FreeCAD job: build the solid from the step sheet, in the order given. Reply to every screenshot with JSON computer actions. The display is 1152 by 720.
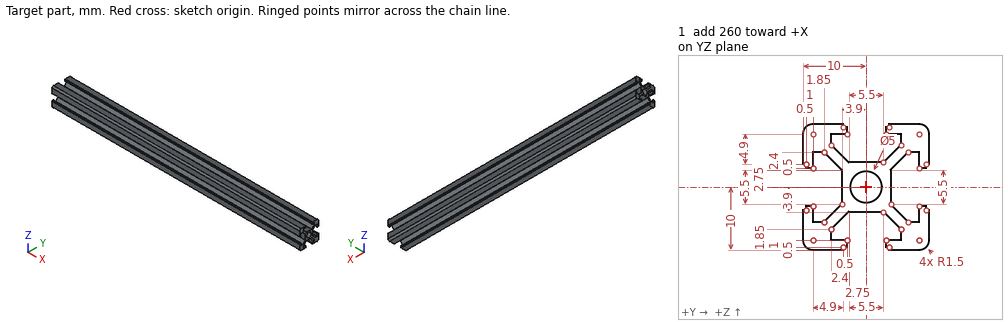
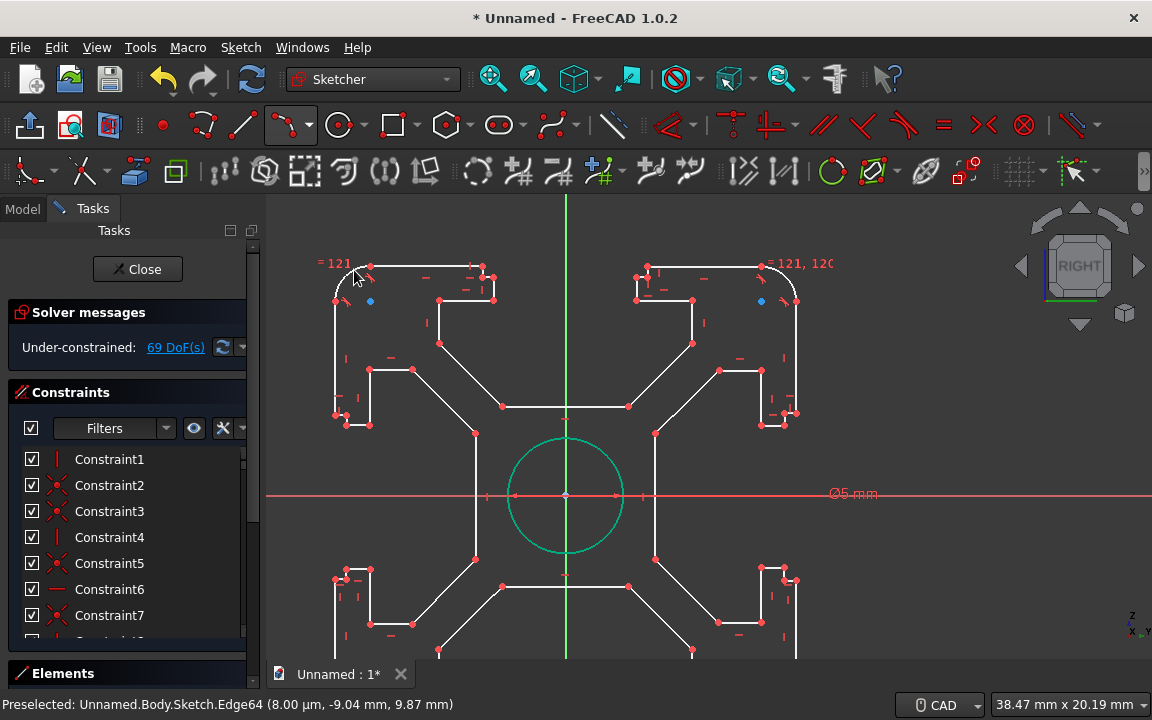
{"action": "scroll", "coordinate": [793, 286], "scroll_direction": "down", "scroll_amount": 2}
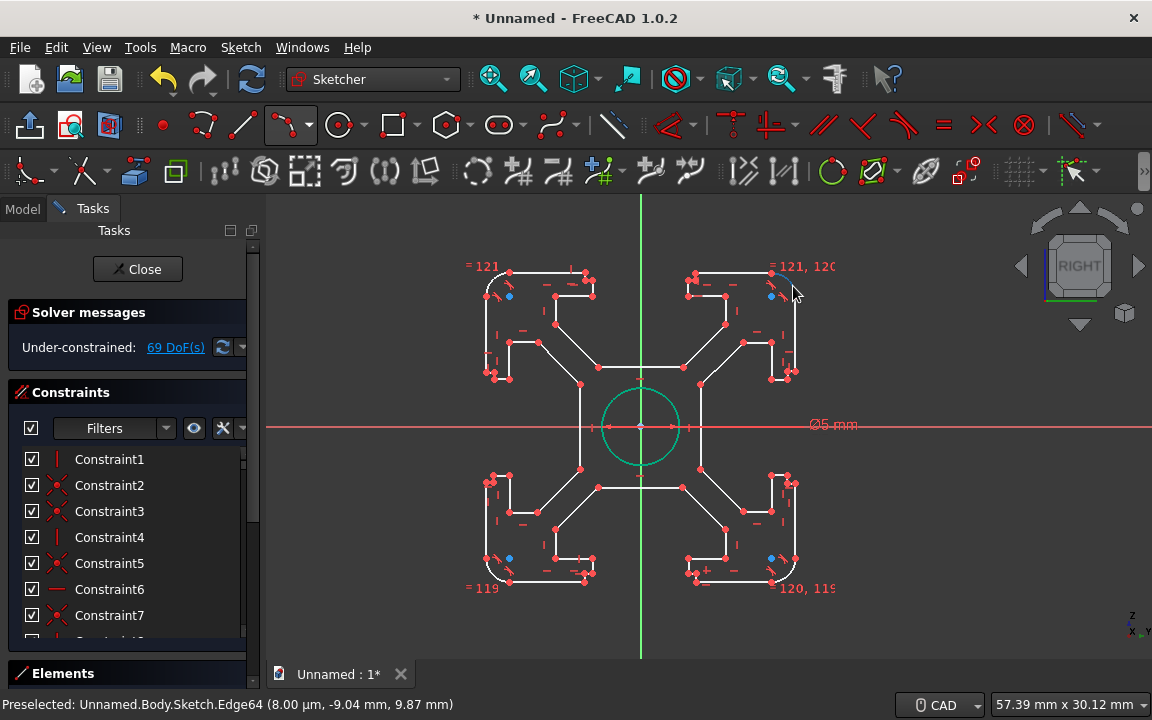
{"action": "left_click", "coordinate": [510, 559]}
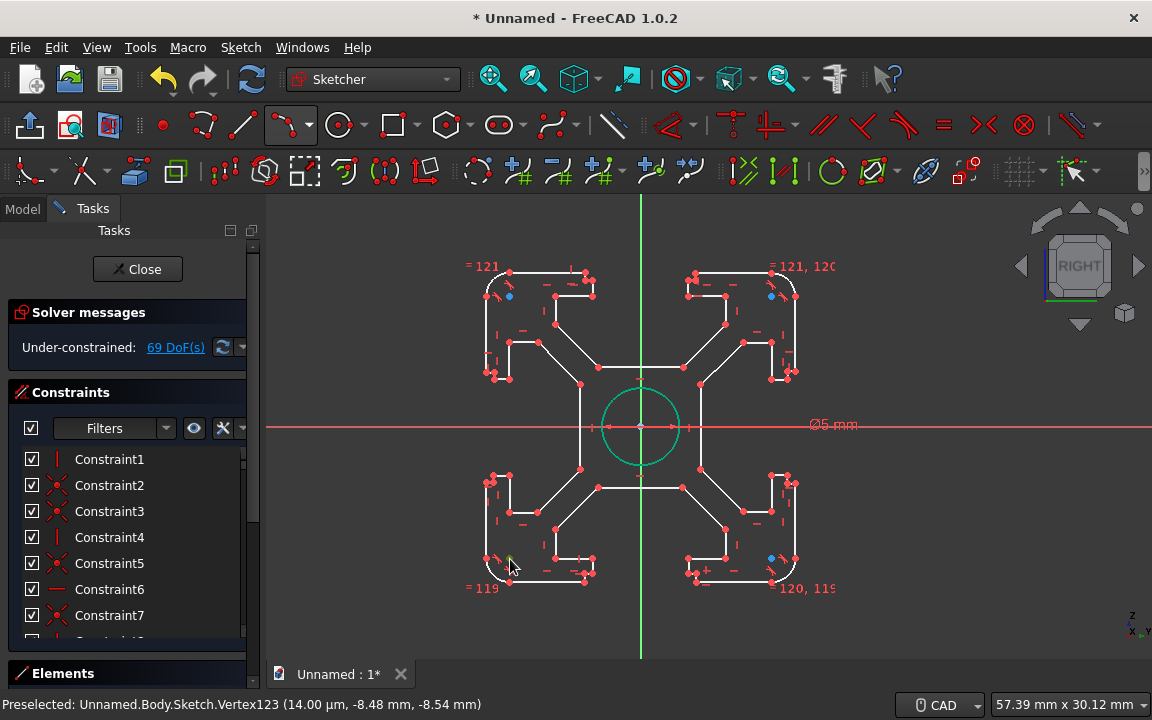
{"action": "left_click", "coordinate": [772, 559]}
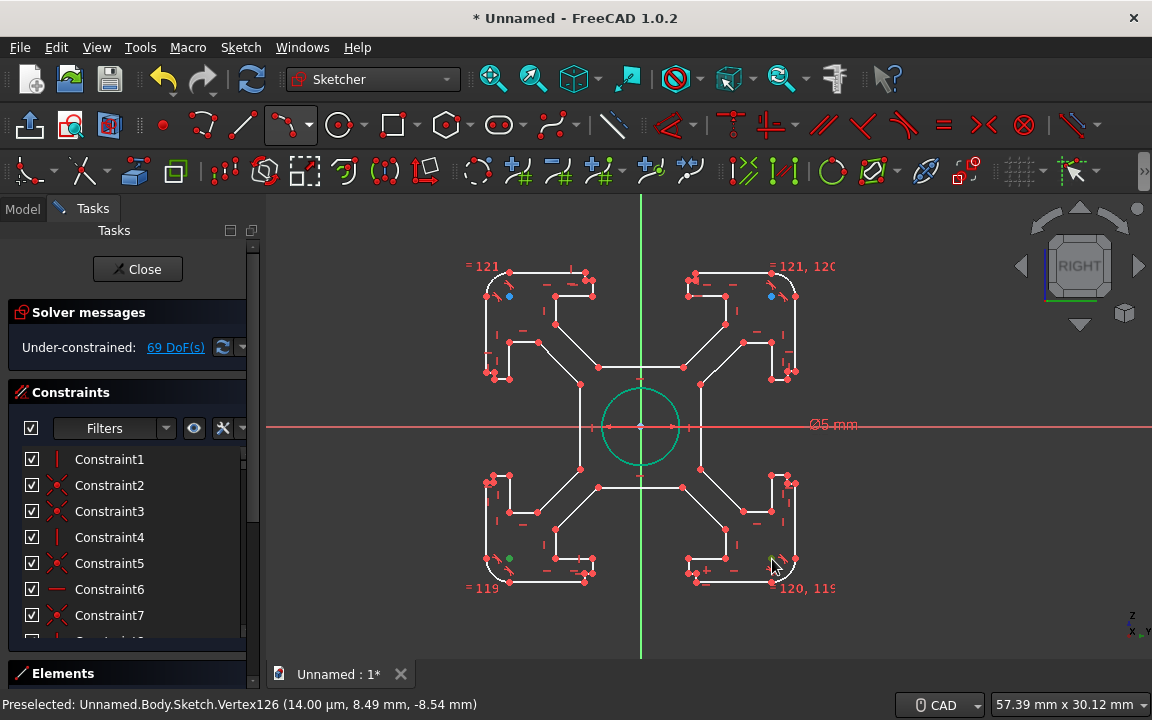
{"action": "left_click", "coordinate": [641, 602]}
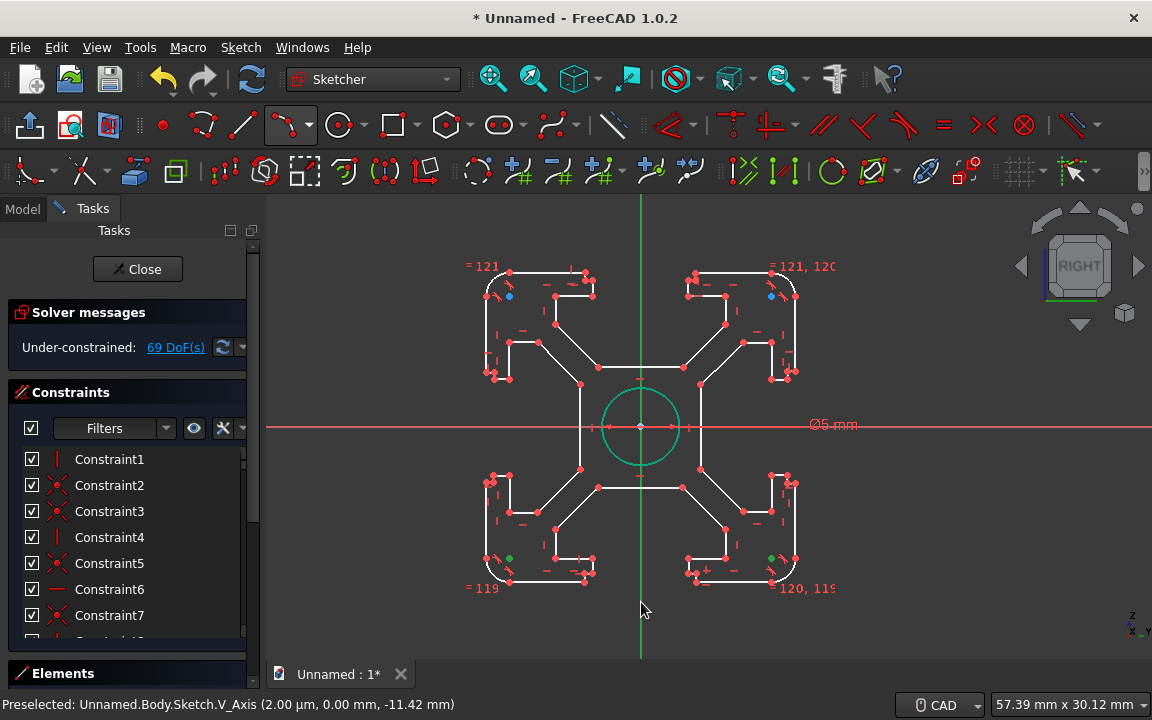
{"action": "left_click", "coordinate": [984, 126]}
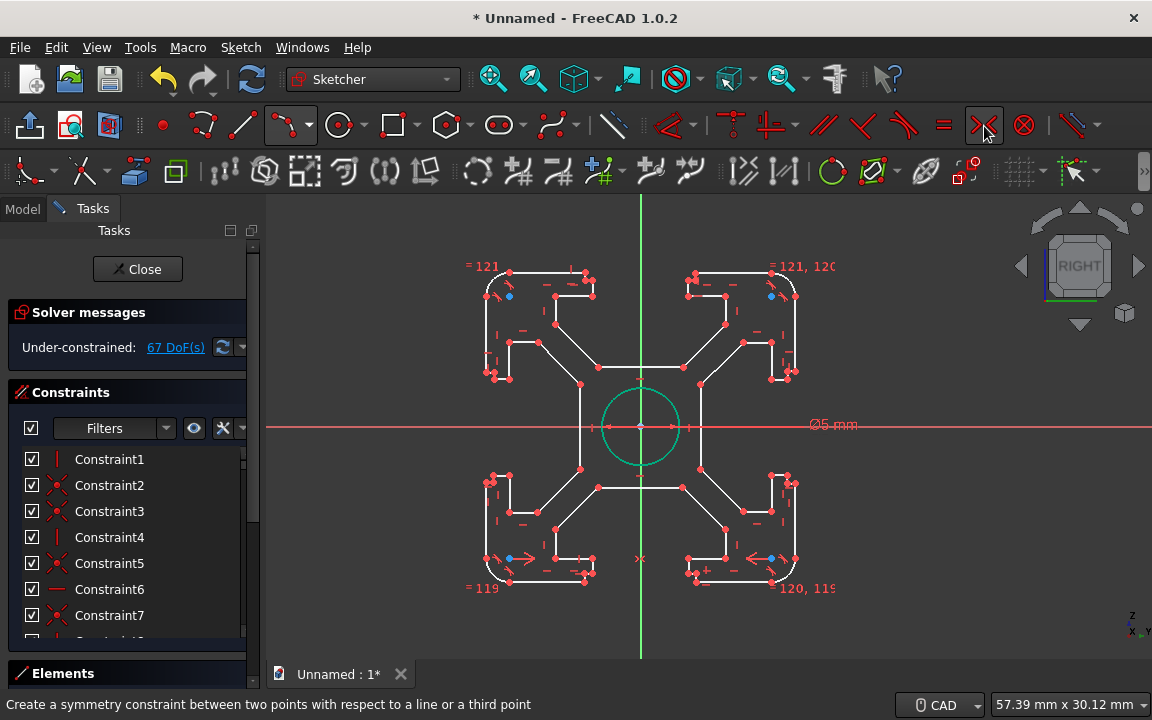
{"action": "left_click", "coordinate": [772, 559]}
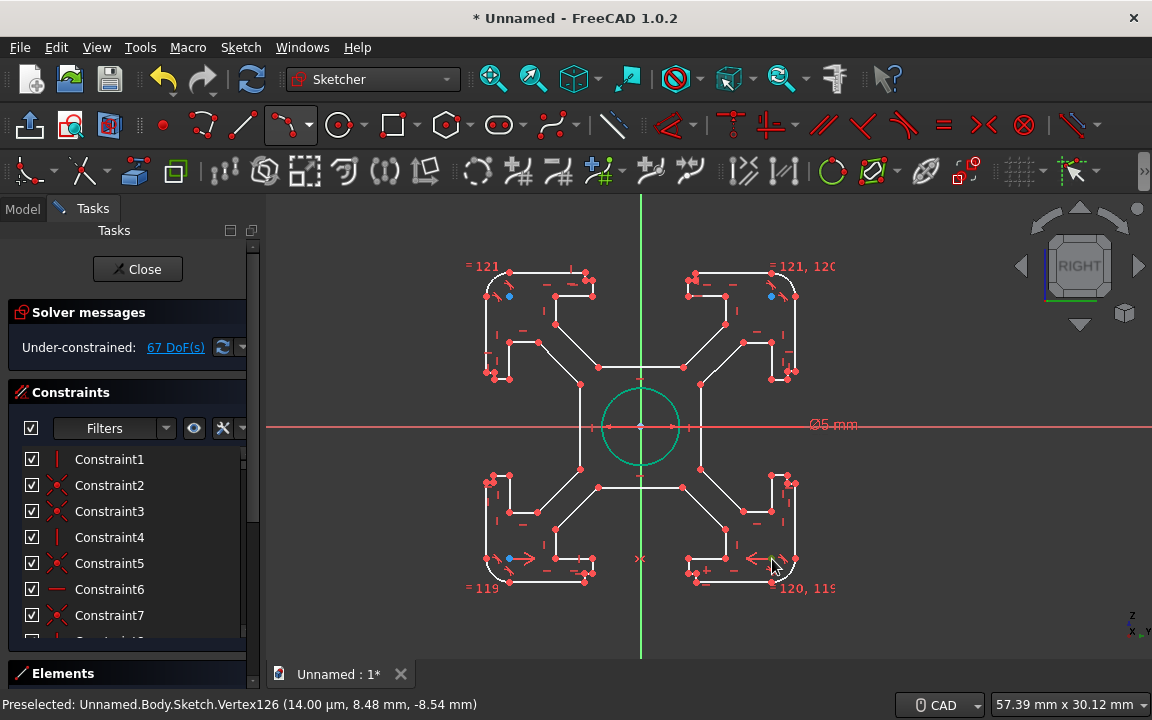
{"action": "left_click", "coordinate": [772, 297]}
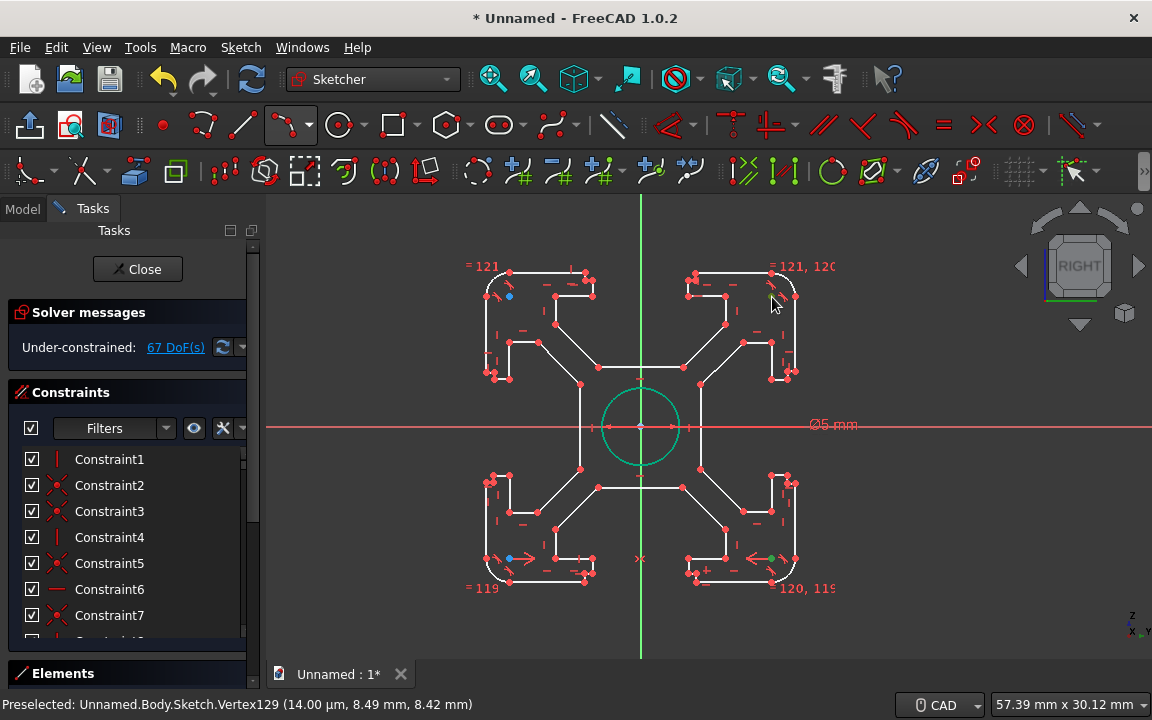
{"action": "left_click", "coordinate": [344, 427]}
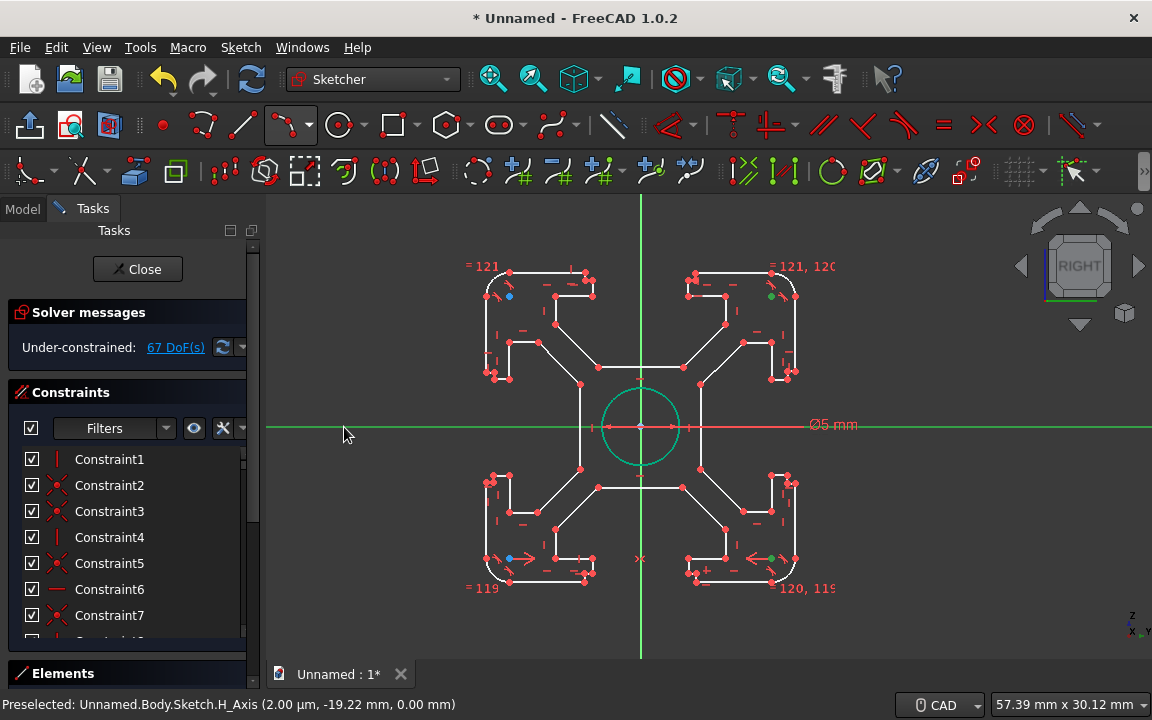
{"action": "key", "text": "s"}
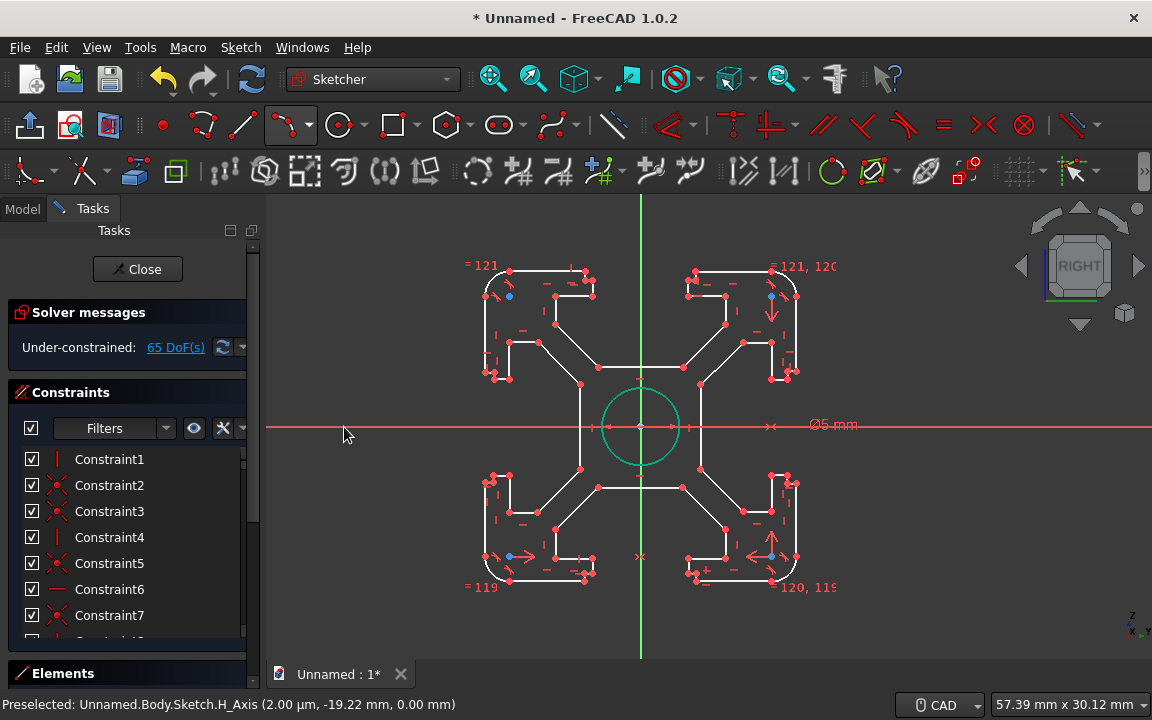
{"action": "left_click", "coordinate": [510, 557]}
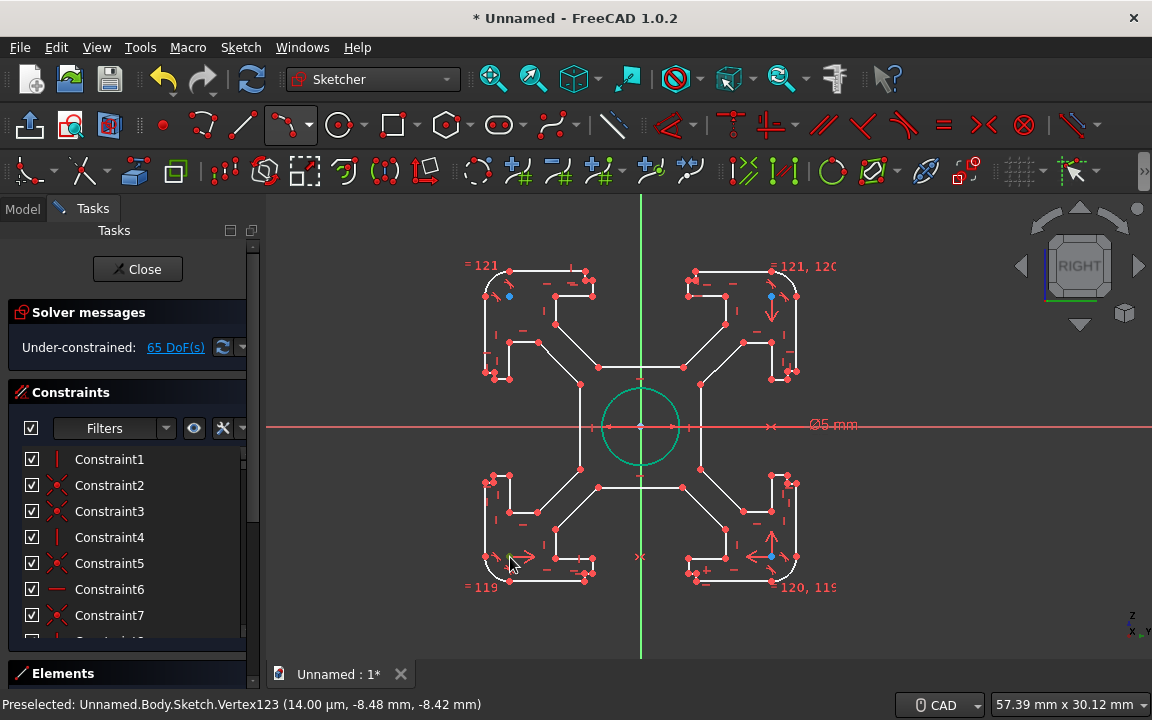
{"action": "left_click", "coordinate": [510, 296]}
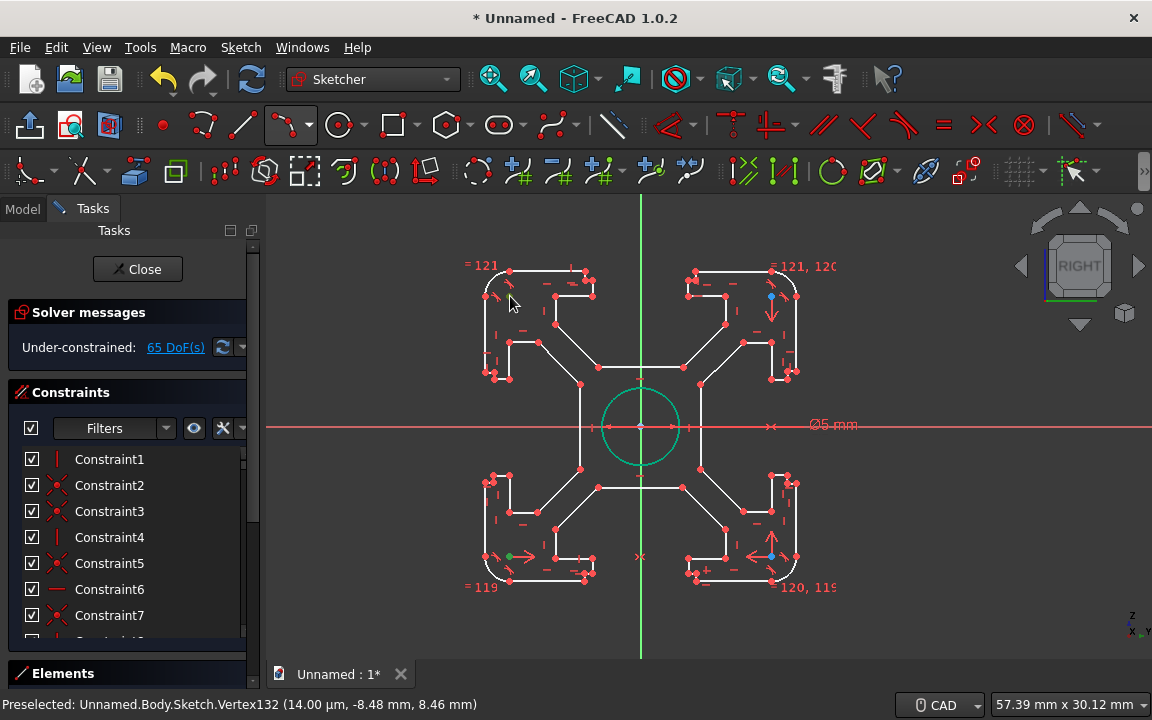
{"action": "left_click", "coordinate": [344, 427]}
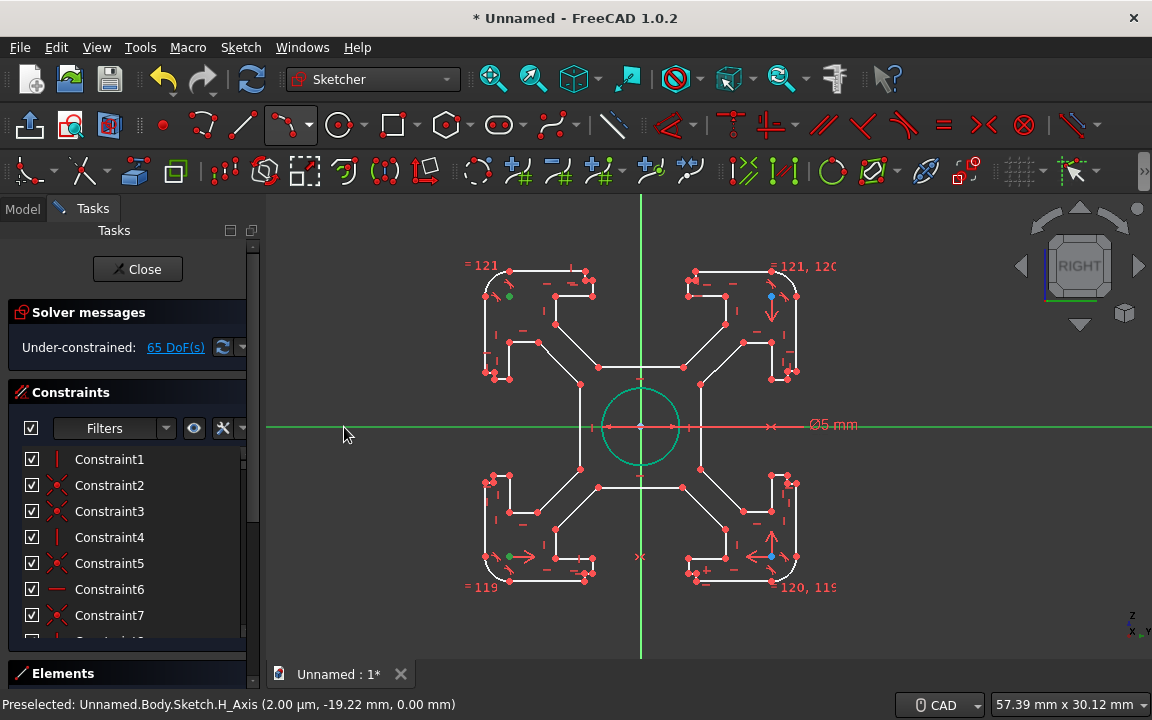
{"action": "left_click", "coordinate": [984, 126]}